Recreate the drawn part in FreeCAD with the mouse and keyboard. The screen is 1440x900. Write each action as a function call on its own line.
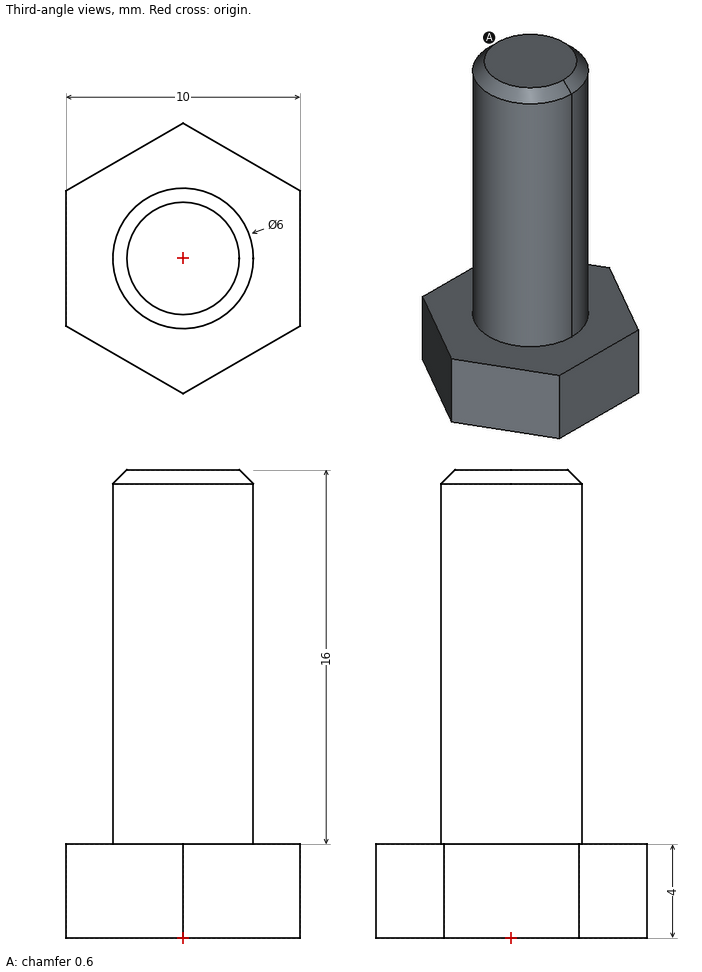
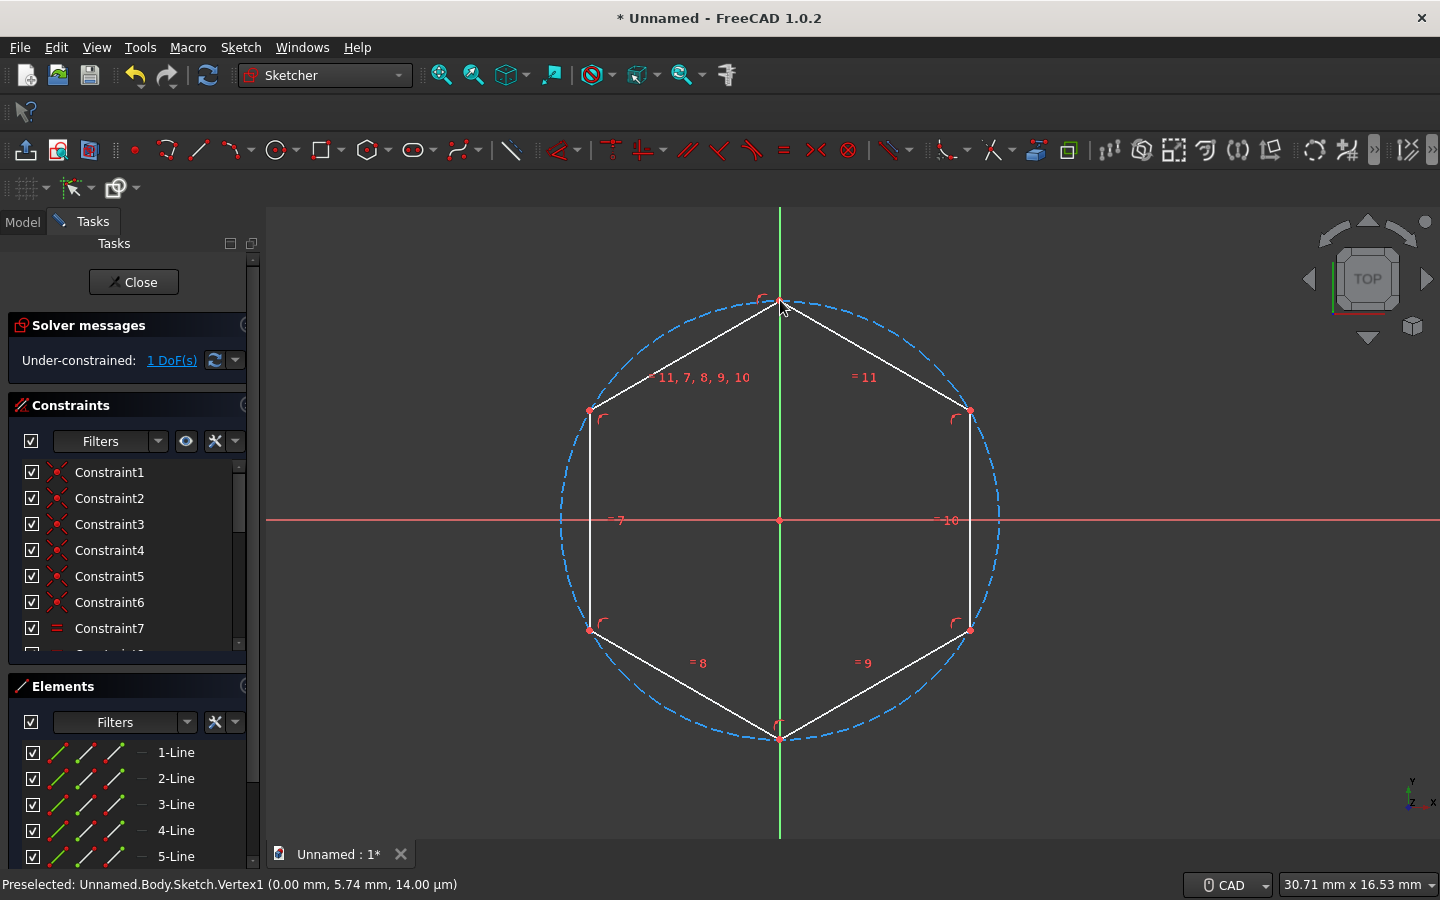
click(558, 150)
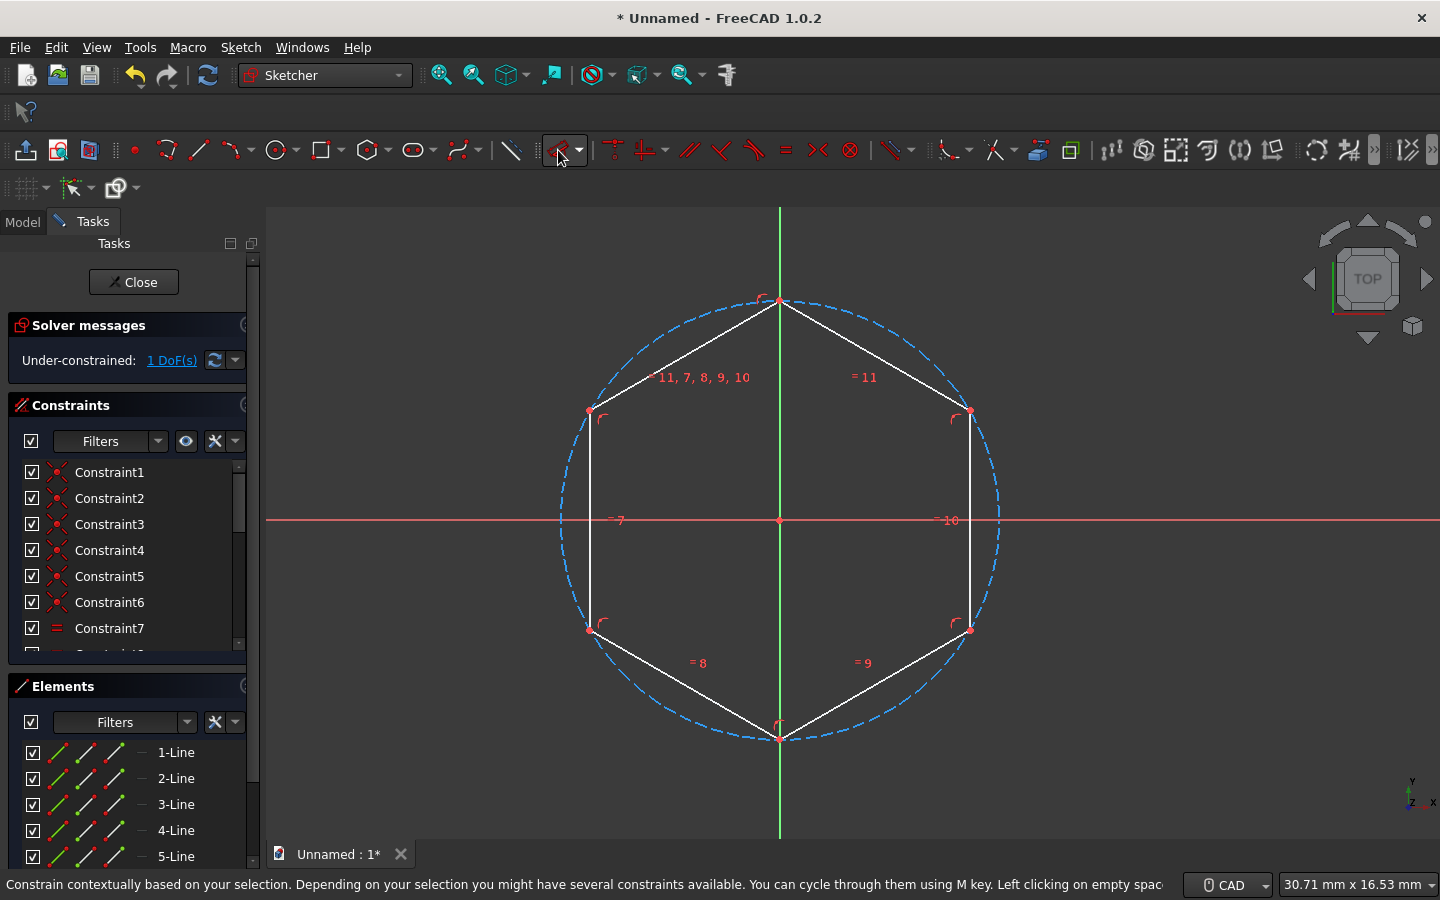
click(590, 411)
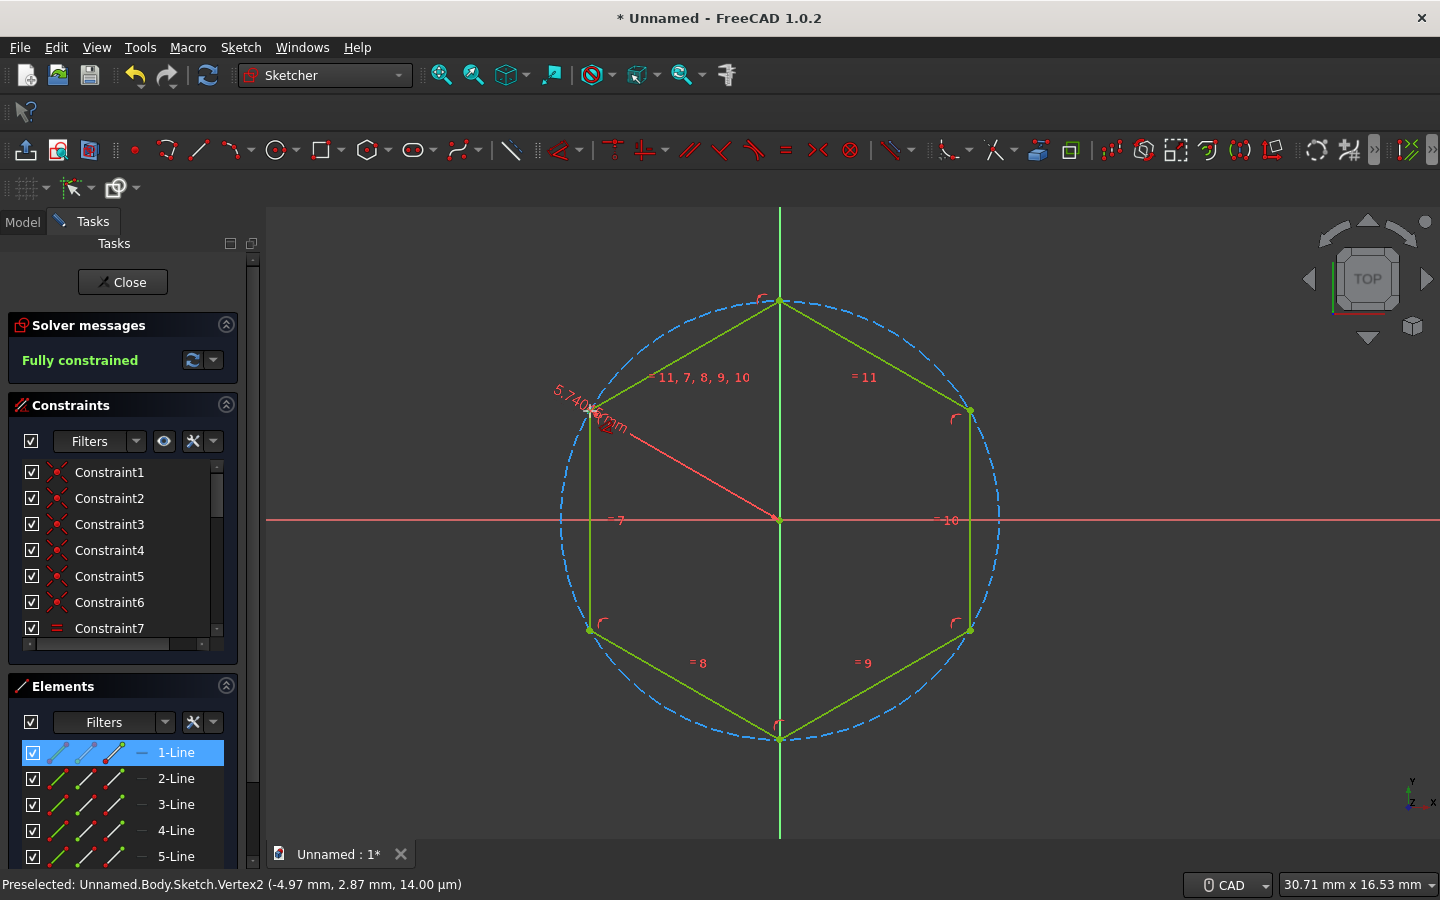
click(970, 630)
click(693, 664)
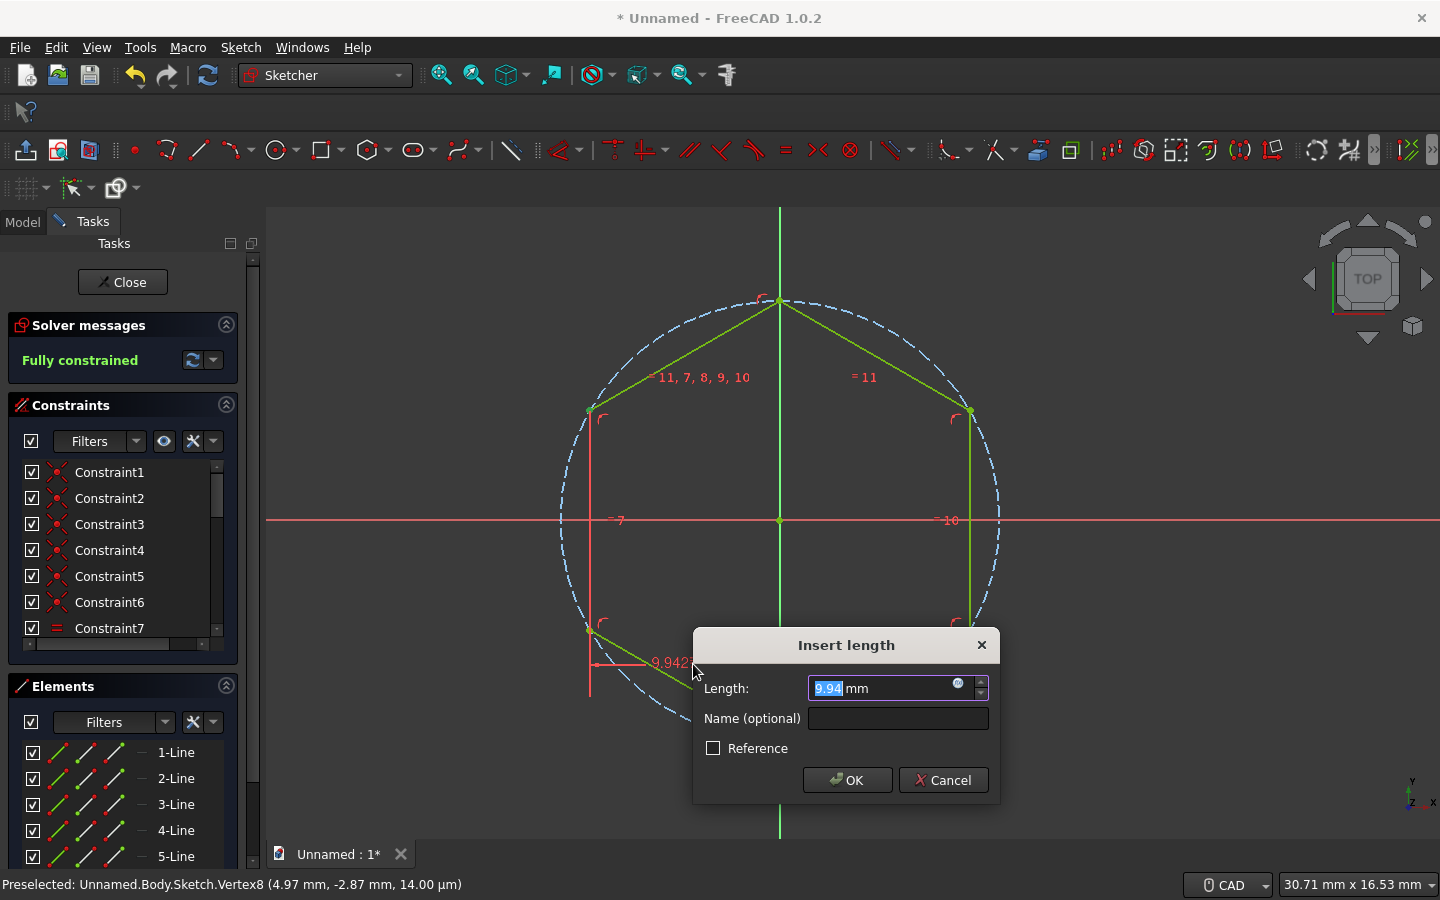
text(10)
key(Return)
key(Escape)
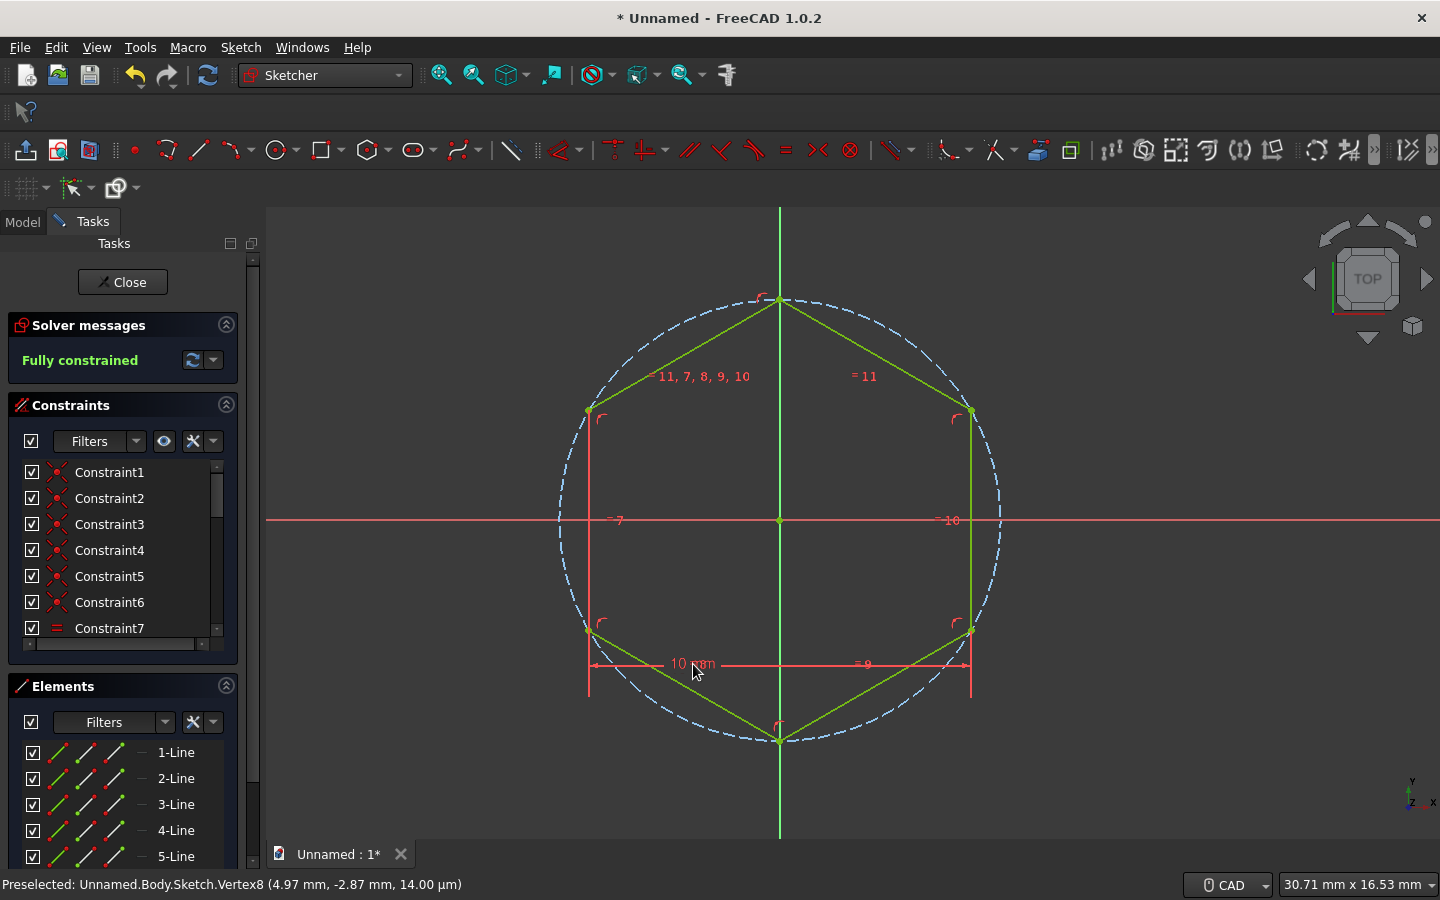
click(123, 282)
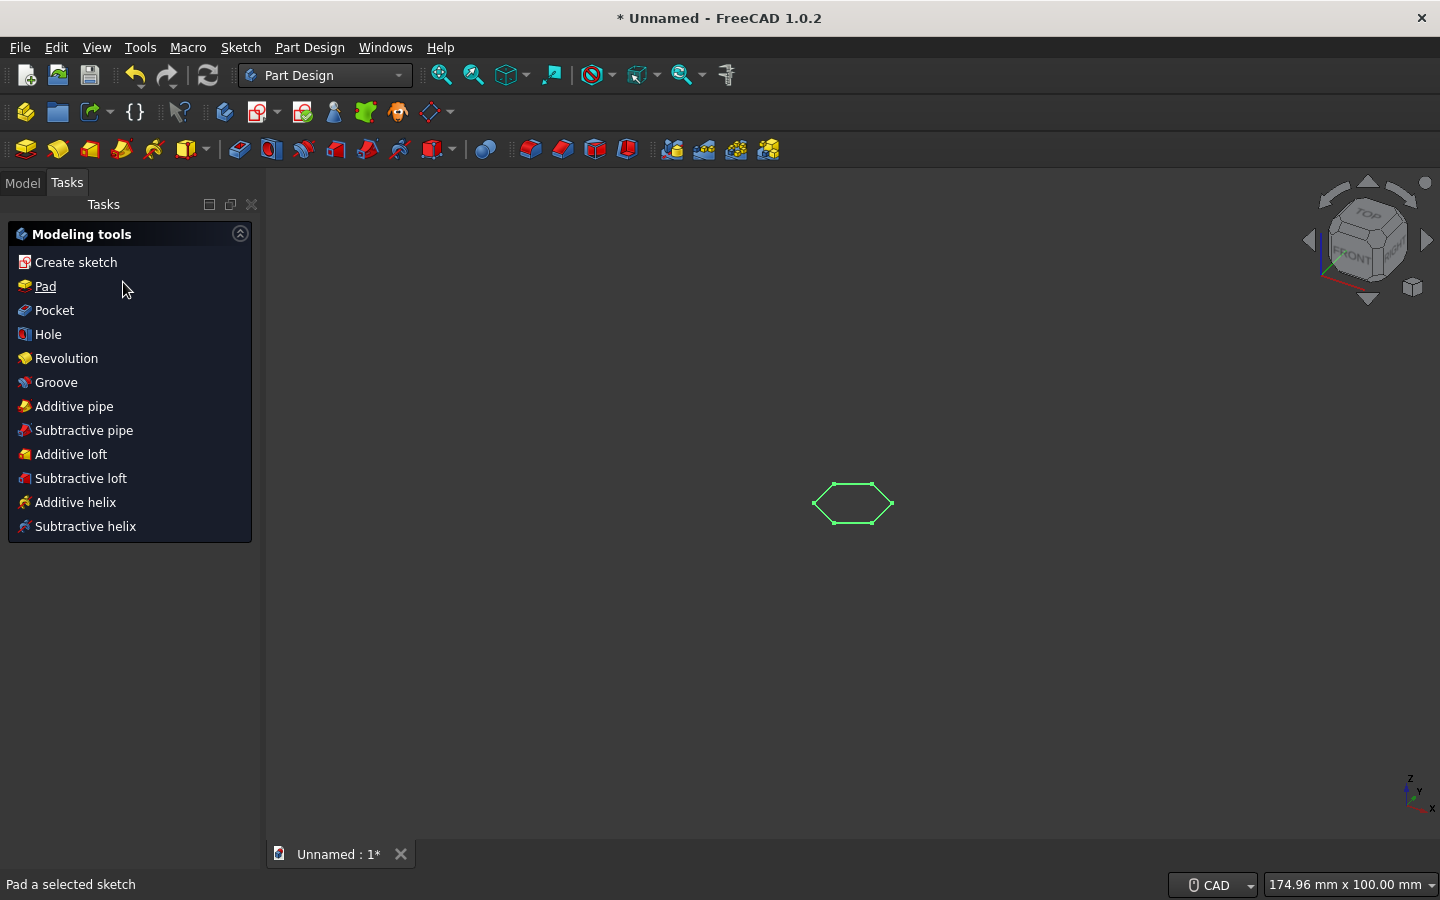
click(26, 150)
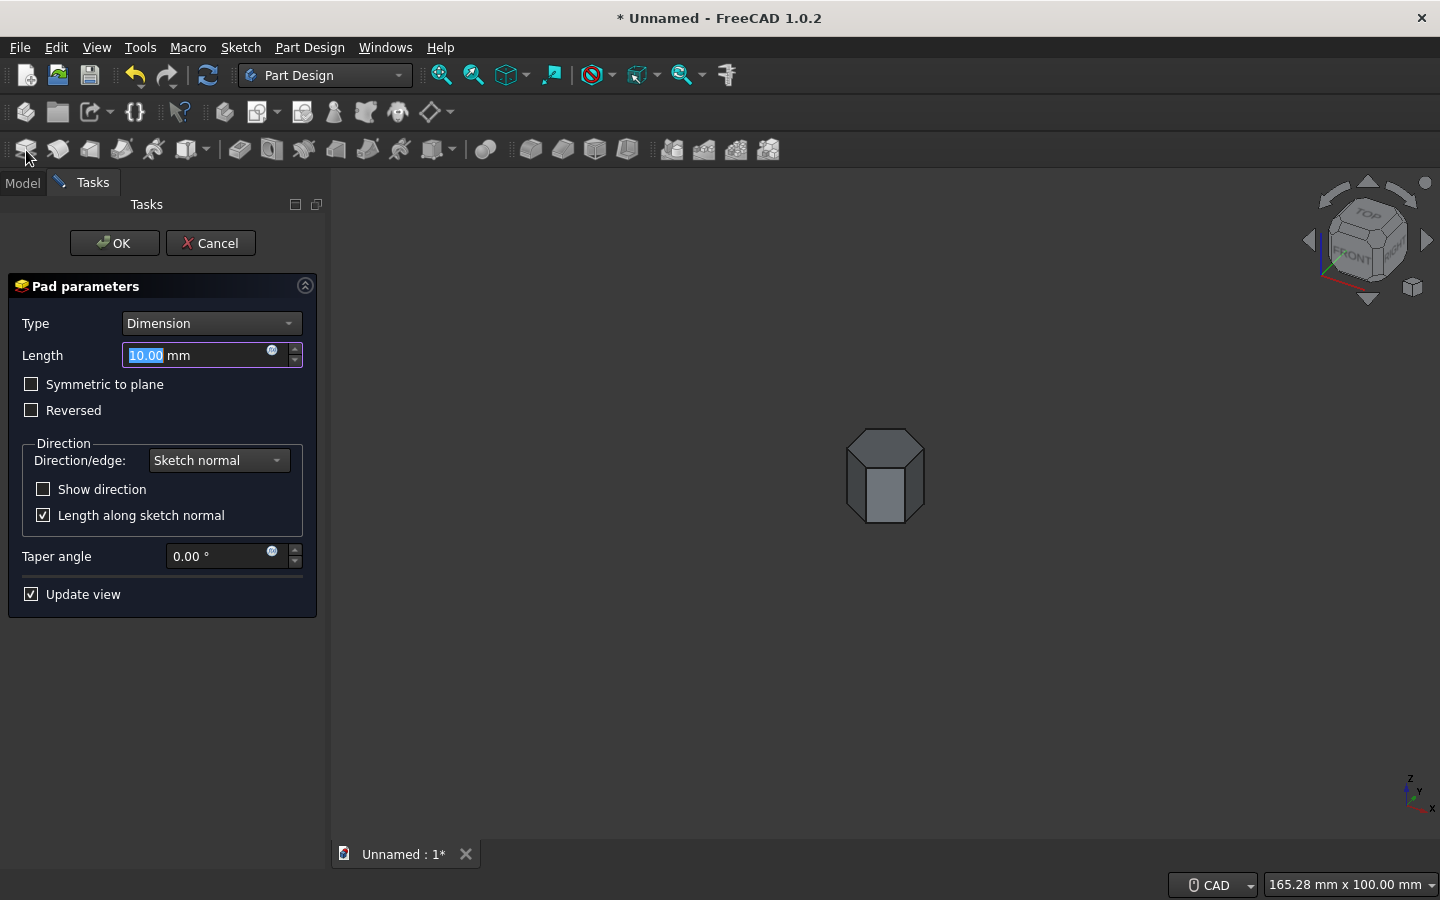
text(4)
key(Tab)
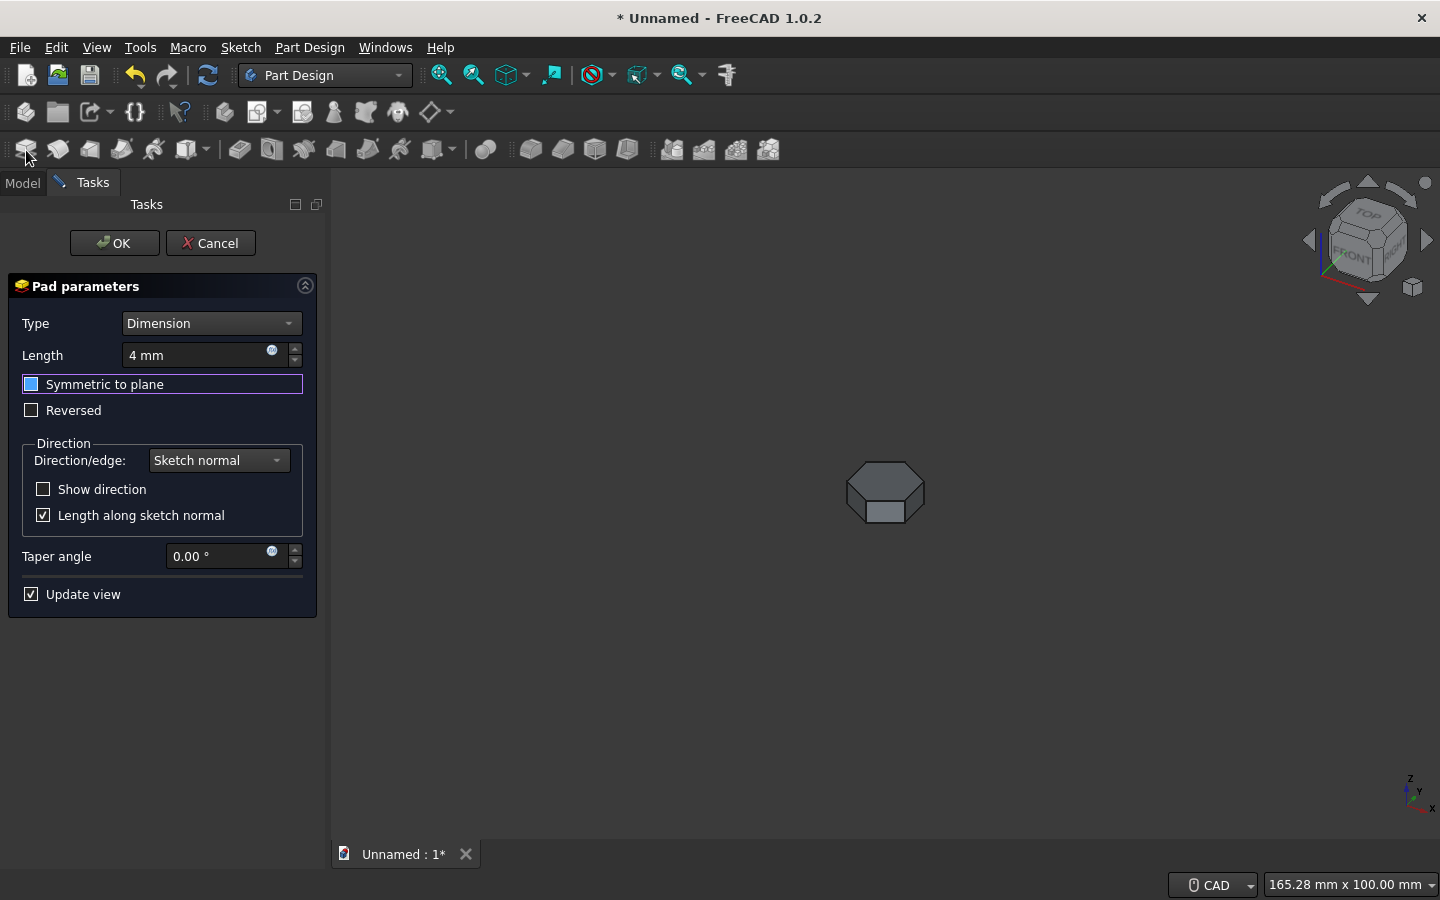
click(115, 243)